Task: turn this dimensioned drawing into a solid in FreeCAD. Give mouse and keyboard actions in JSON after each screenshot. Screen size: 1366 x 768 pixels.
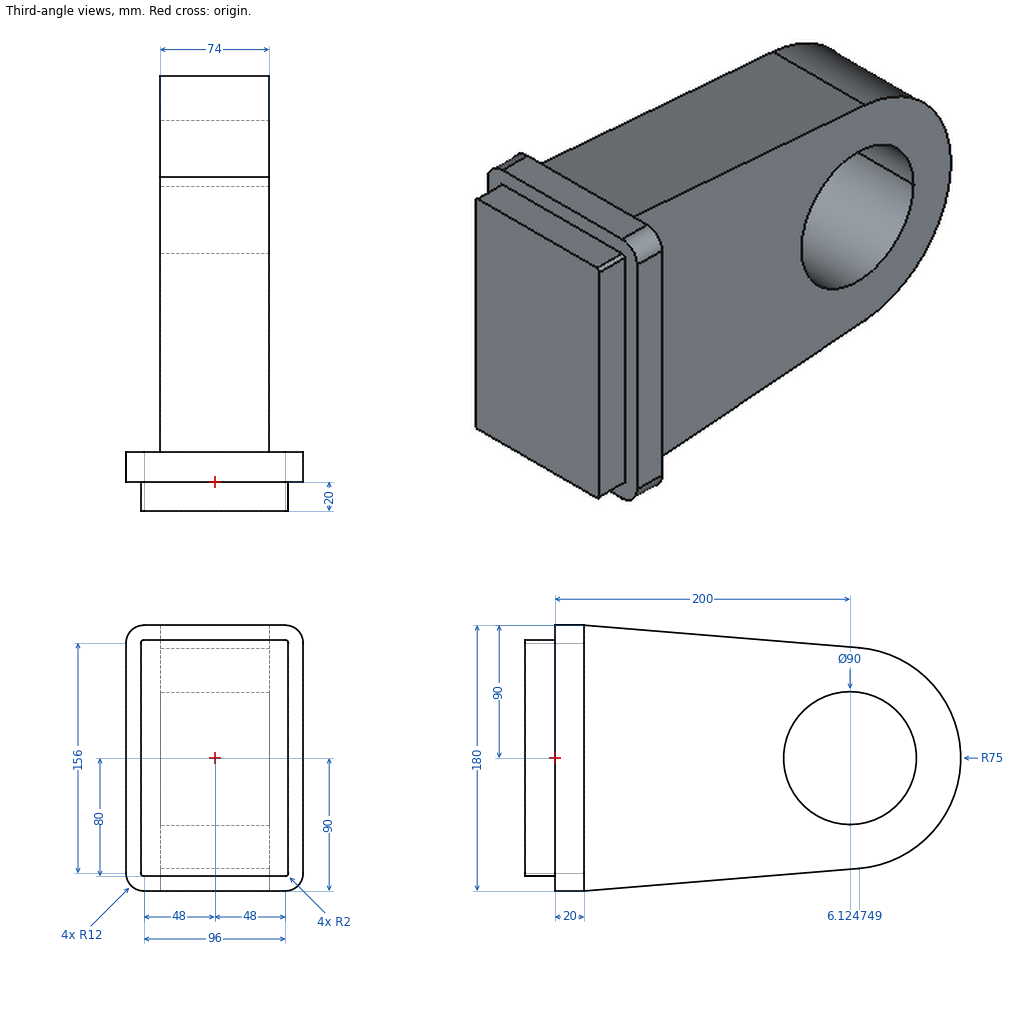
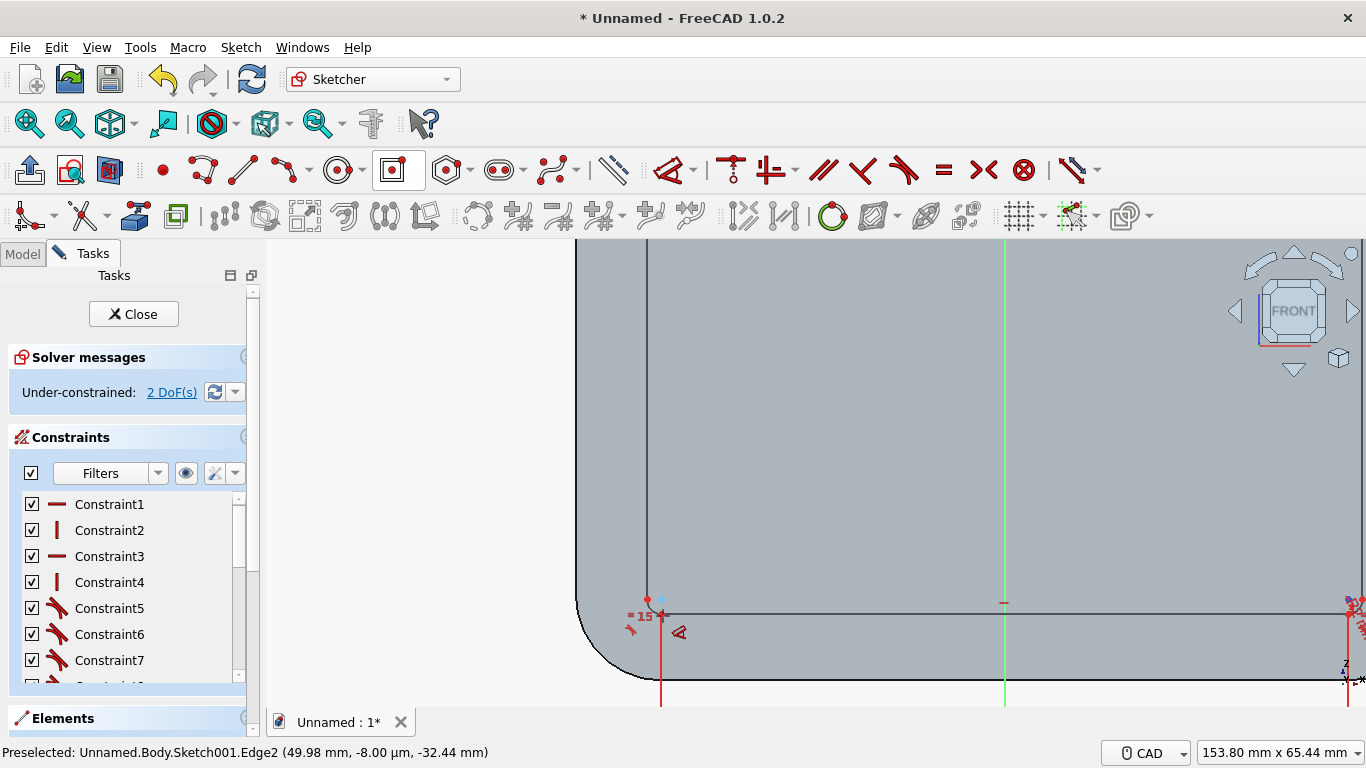
{"action": "left_click", "coordinate": [661, 614]}
{"action": "left_click", "coordinate": [833, 648]}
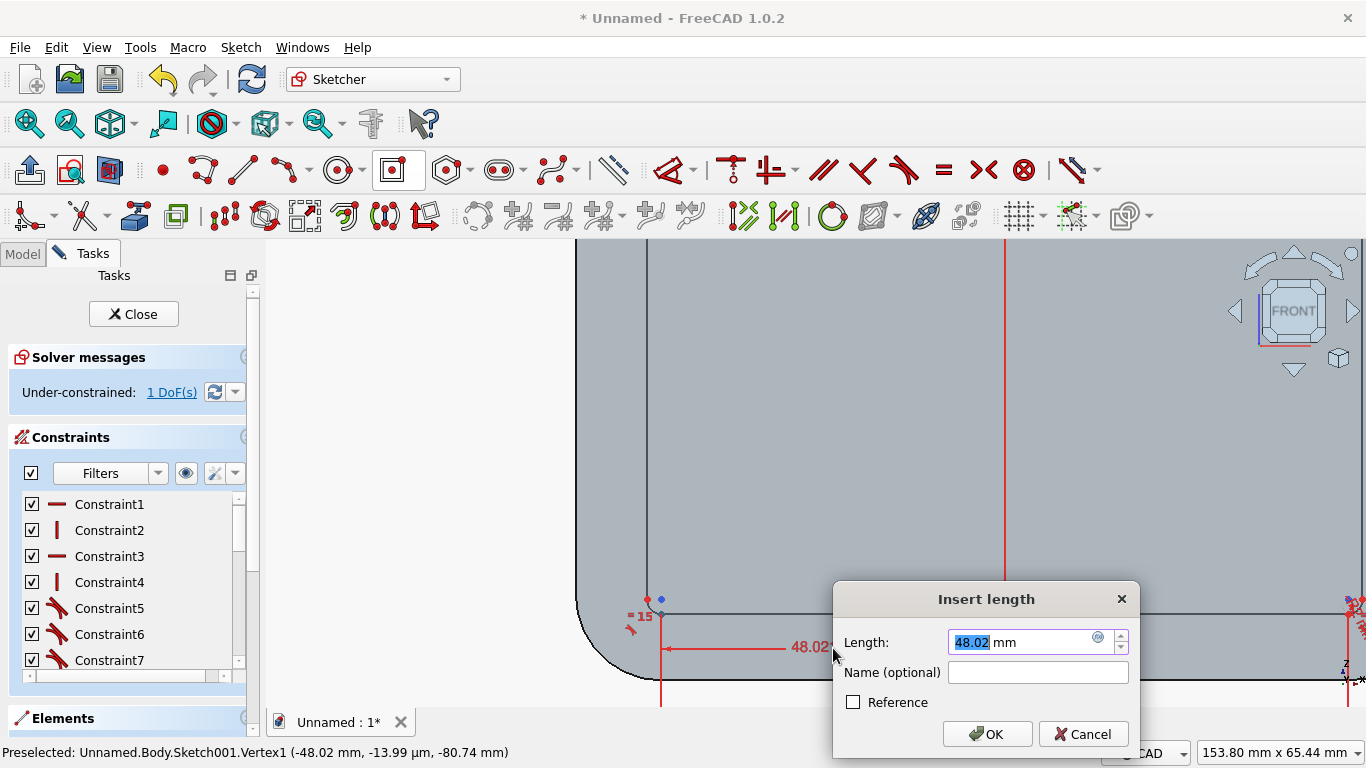
{"action": "type", "text": "48"}
{"action": "key", "text": "Return"}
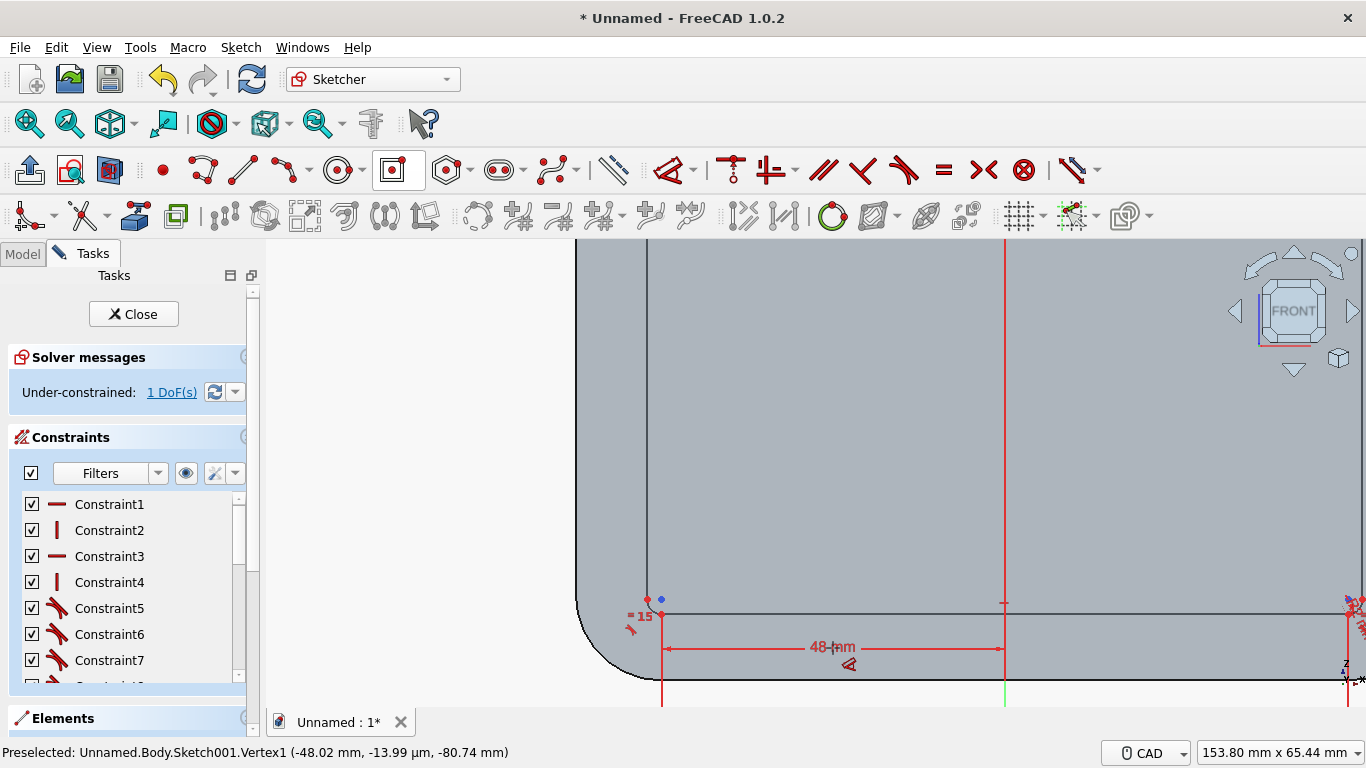
{"action": "left_click", "coordinate": [662, 614]}
{"action": "left_click", "coordinate": [628, 441]}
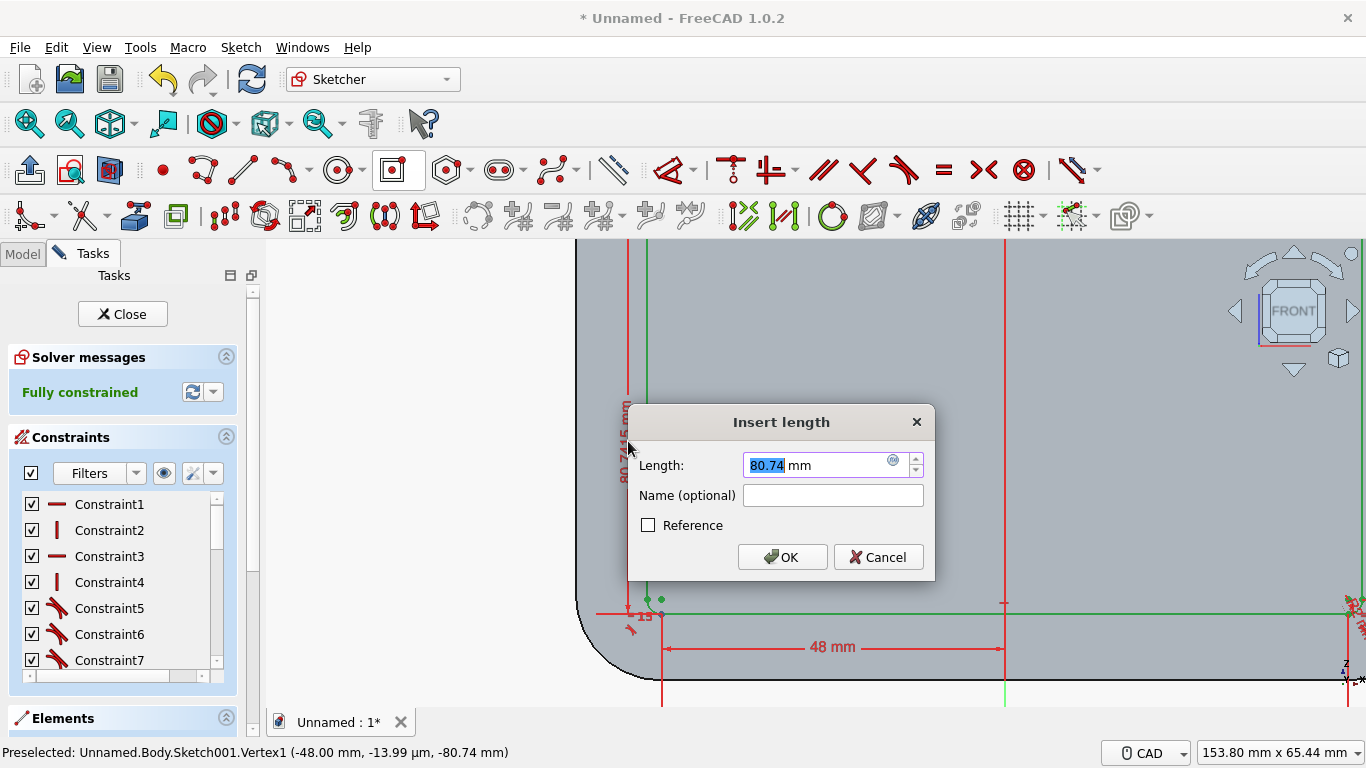
{"action": "type", "text": "80"}
{"action": "key", "text": "Return"}
{"action": "key", "text": "Escape"}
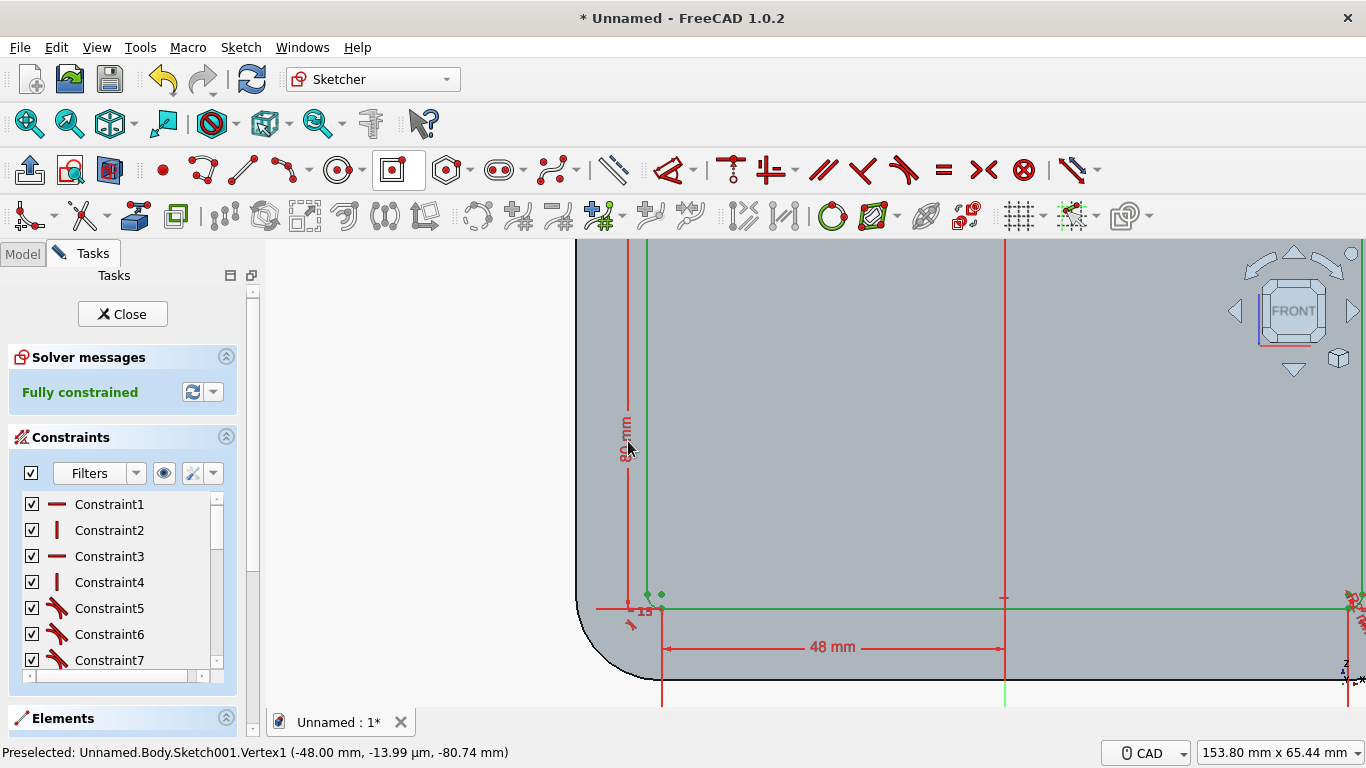
{"action": "left_click", "coordinate": [123, 314]}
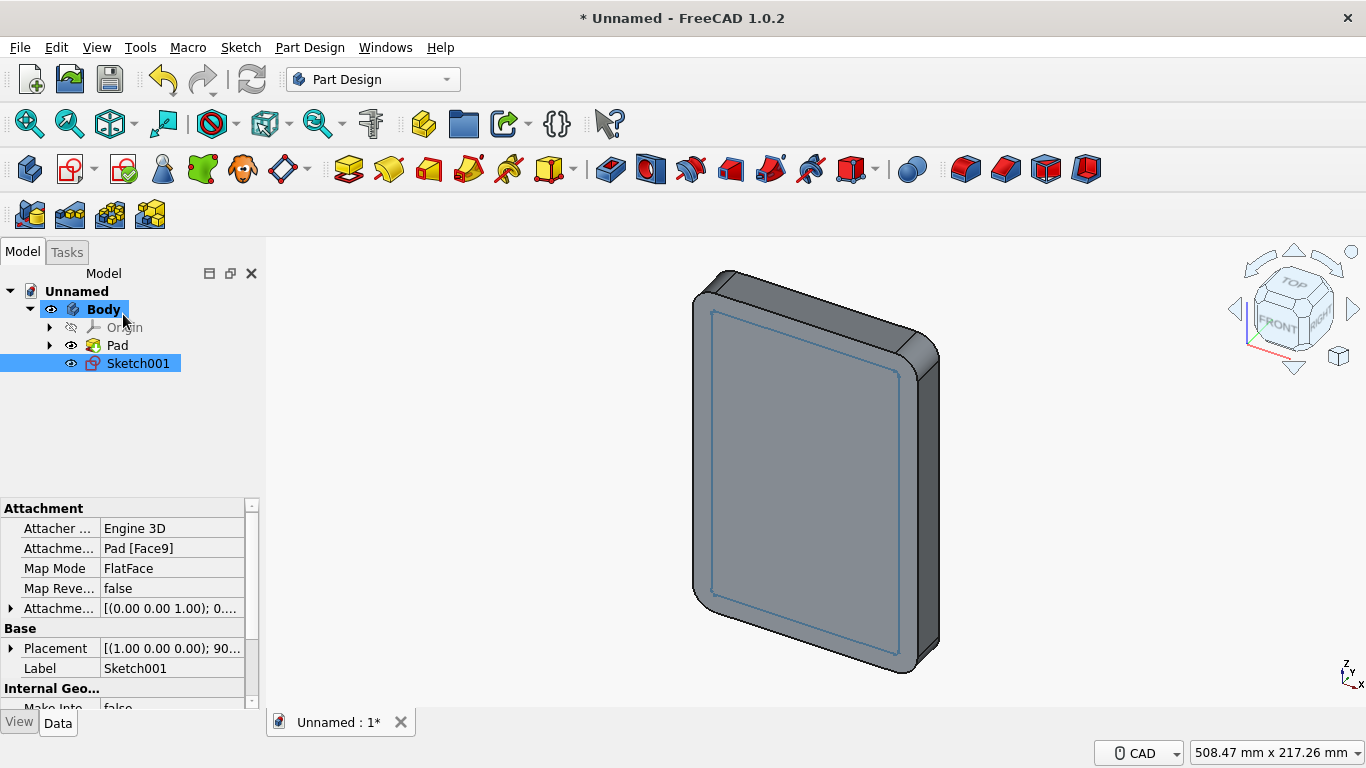
{"action": "left_click", "coordinate": [350, 170]}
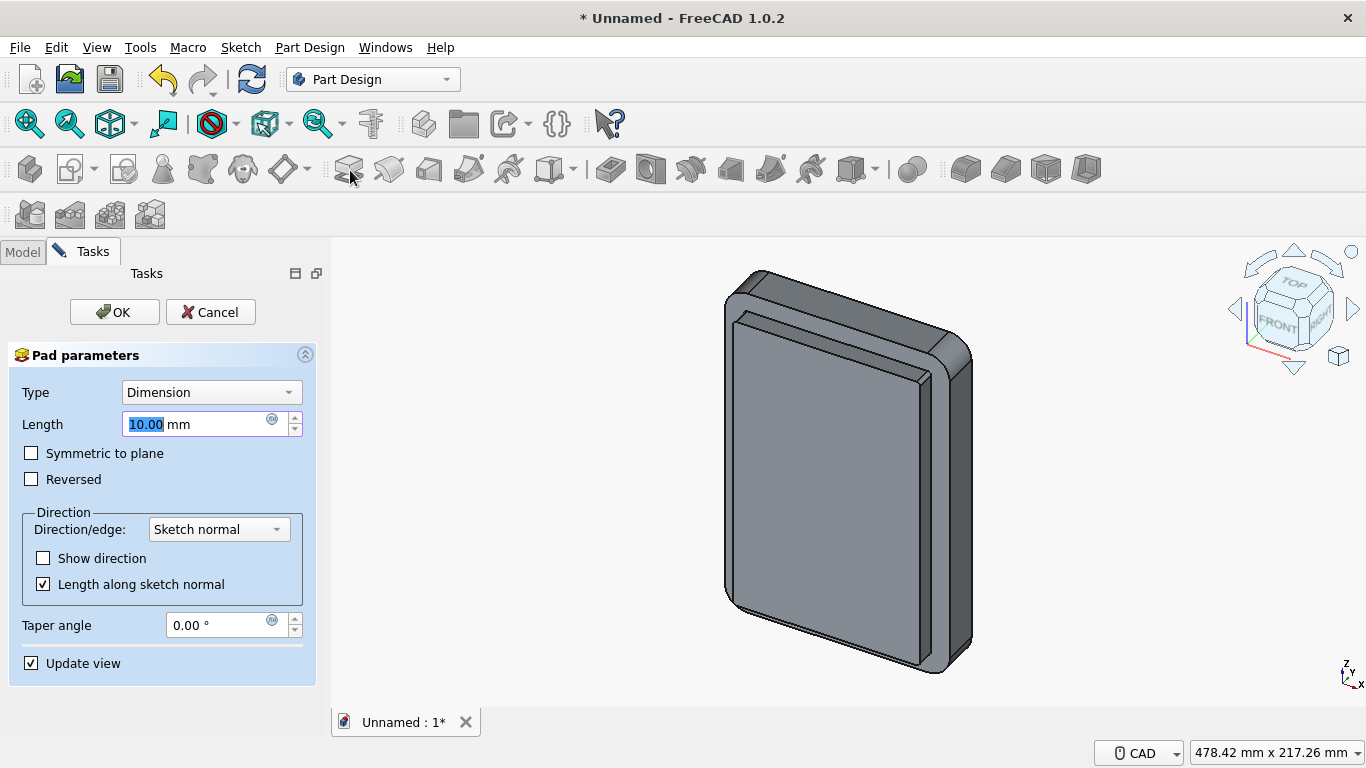
{"action": "type", "text": "20"}
{"action": "key", "text": "Tab"}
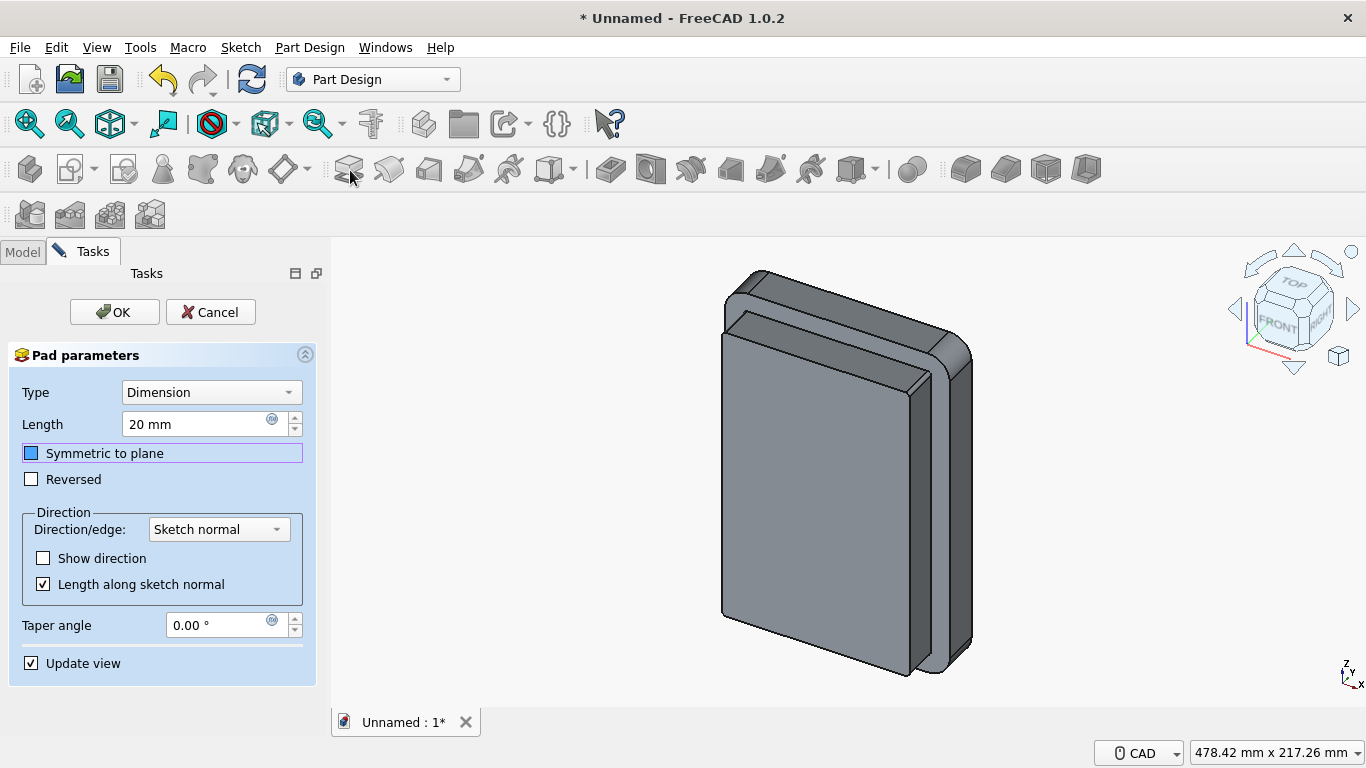
{"action": "left_click", "coordinate": [115, 312]}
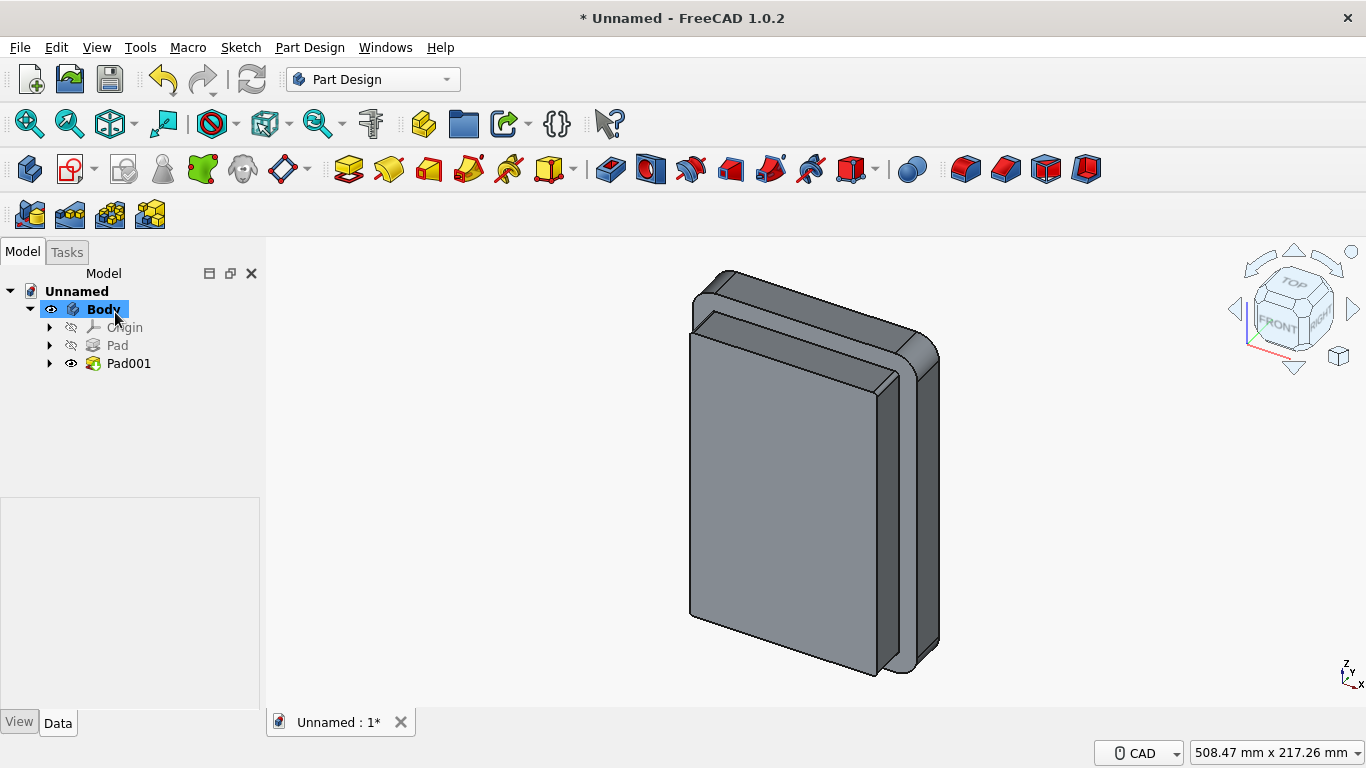
{"action": "left_click", "coordinate": [70, 170]}